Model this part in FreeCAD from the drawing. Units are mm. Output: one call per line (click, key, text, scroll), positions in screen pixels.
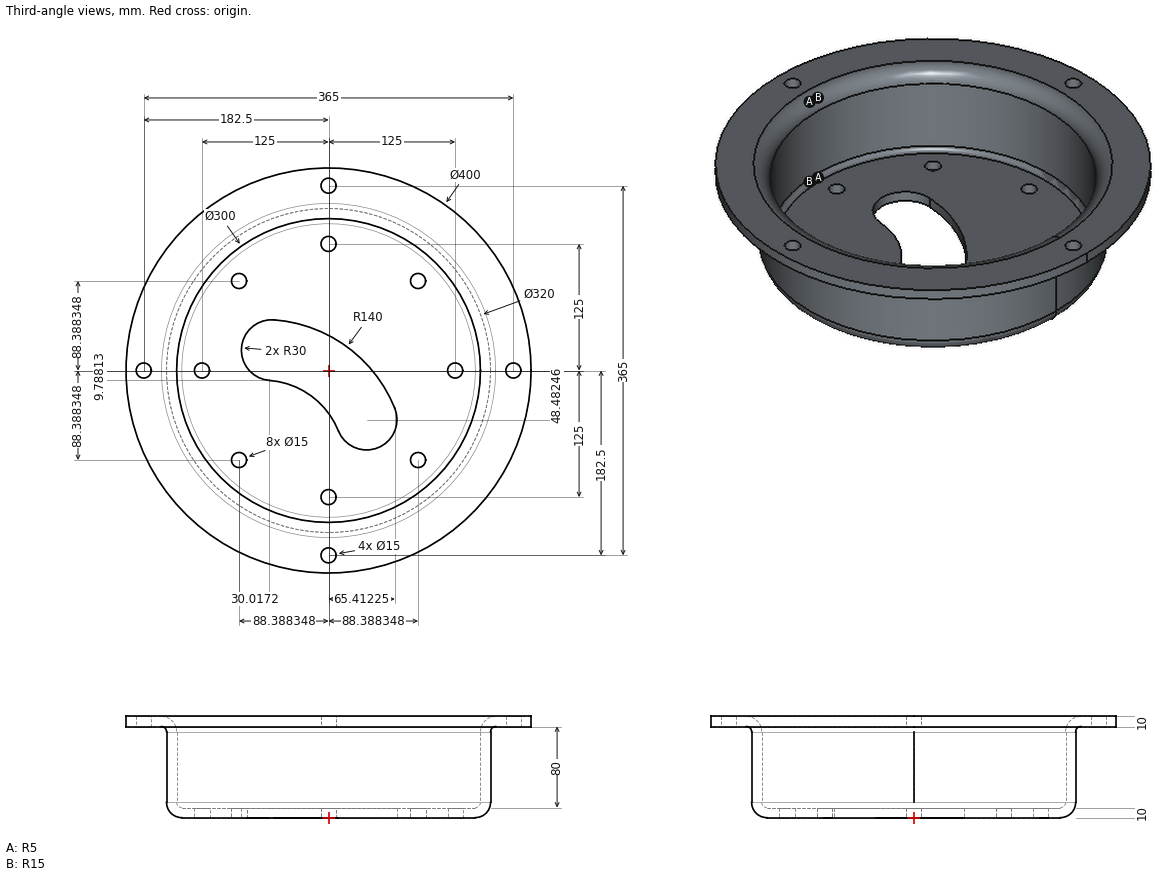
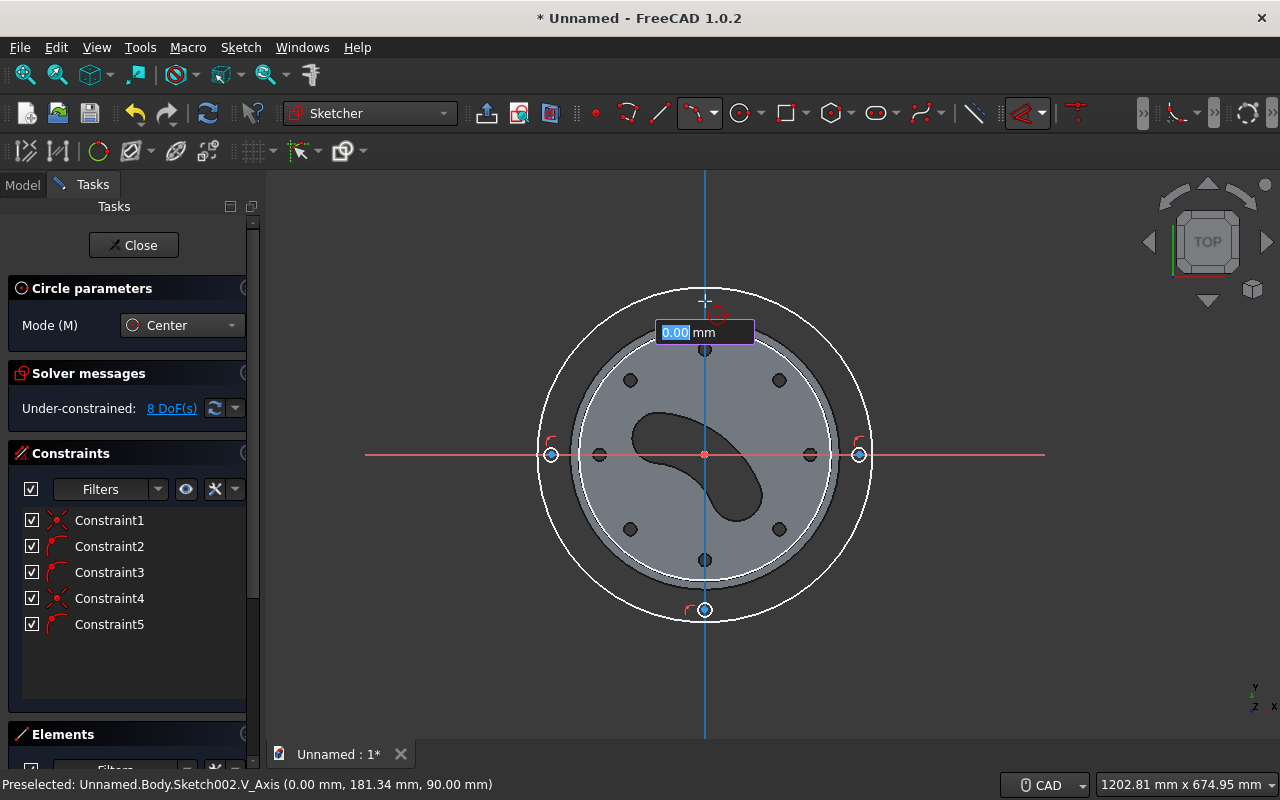
scroll(711, 299, up, 5)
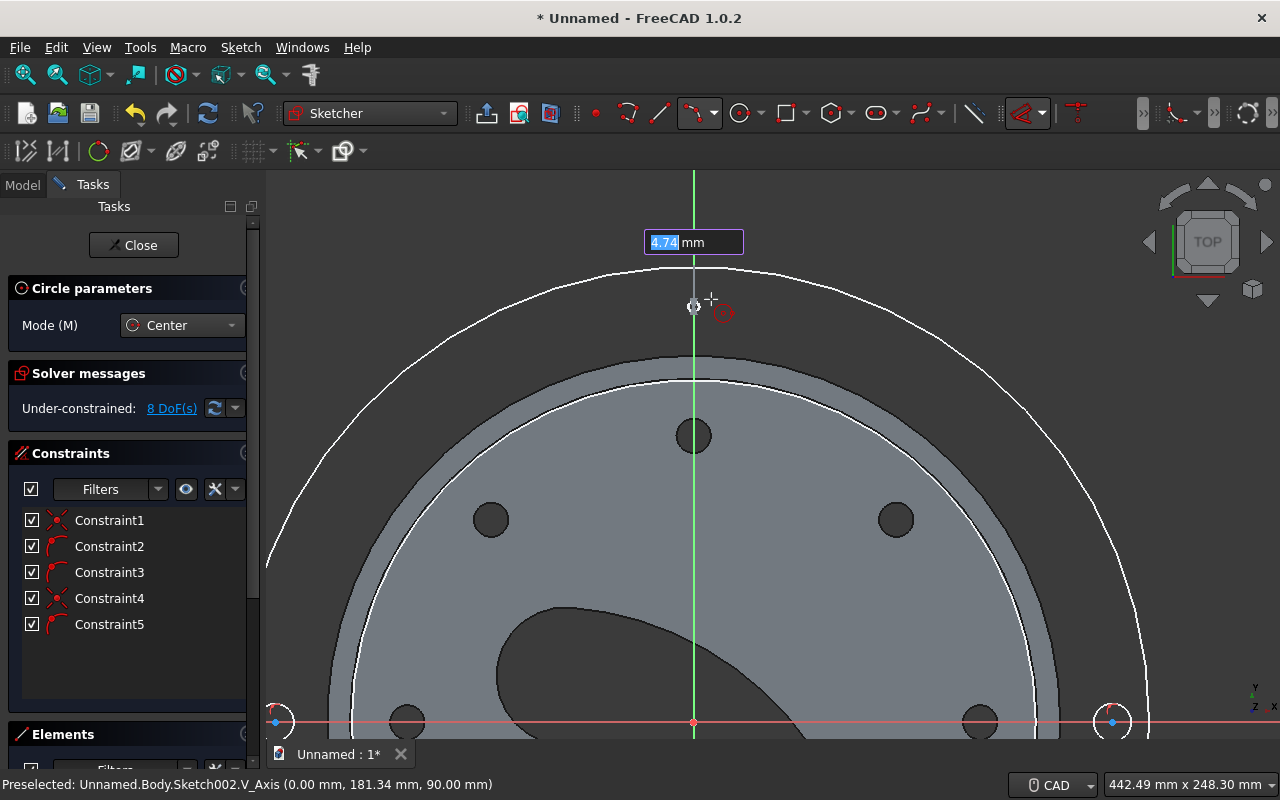
click(710, 298)
key(Escape)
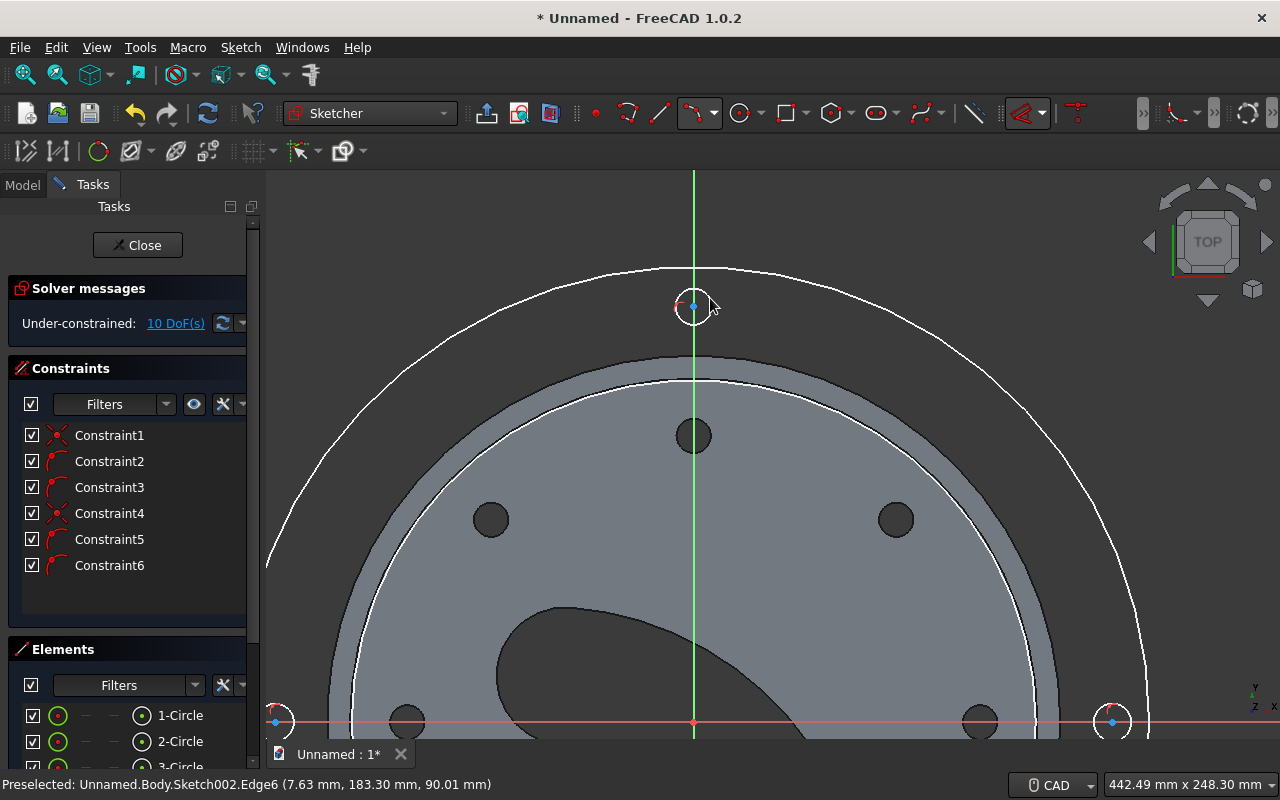
scroll(711, 299, down, 5)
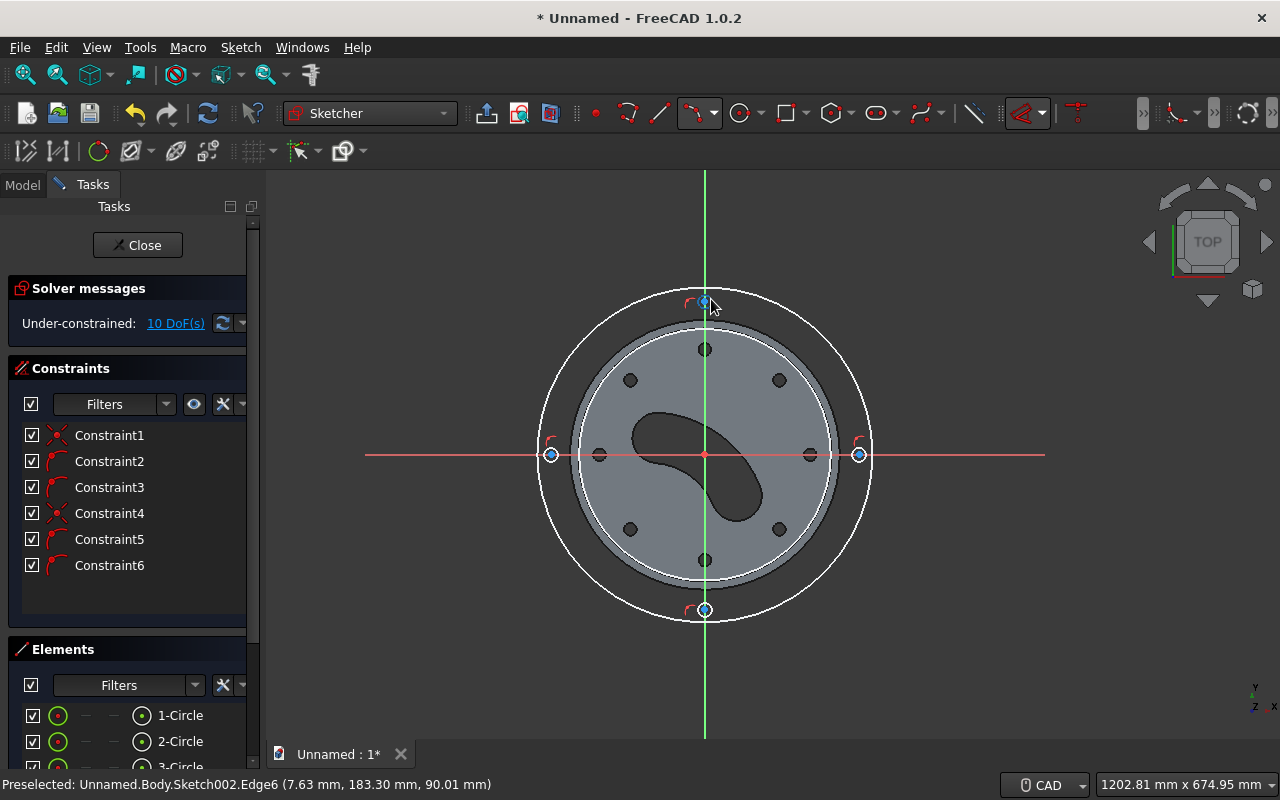
scroll(710, 605, up, 6)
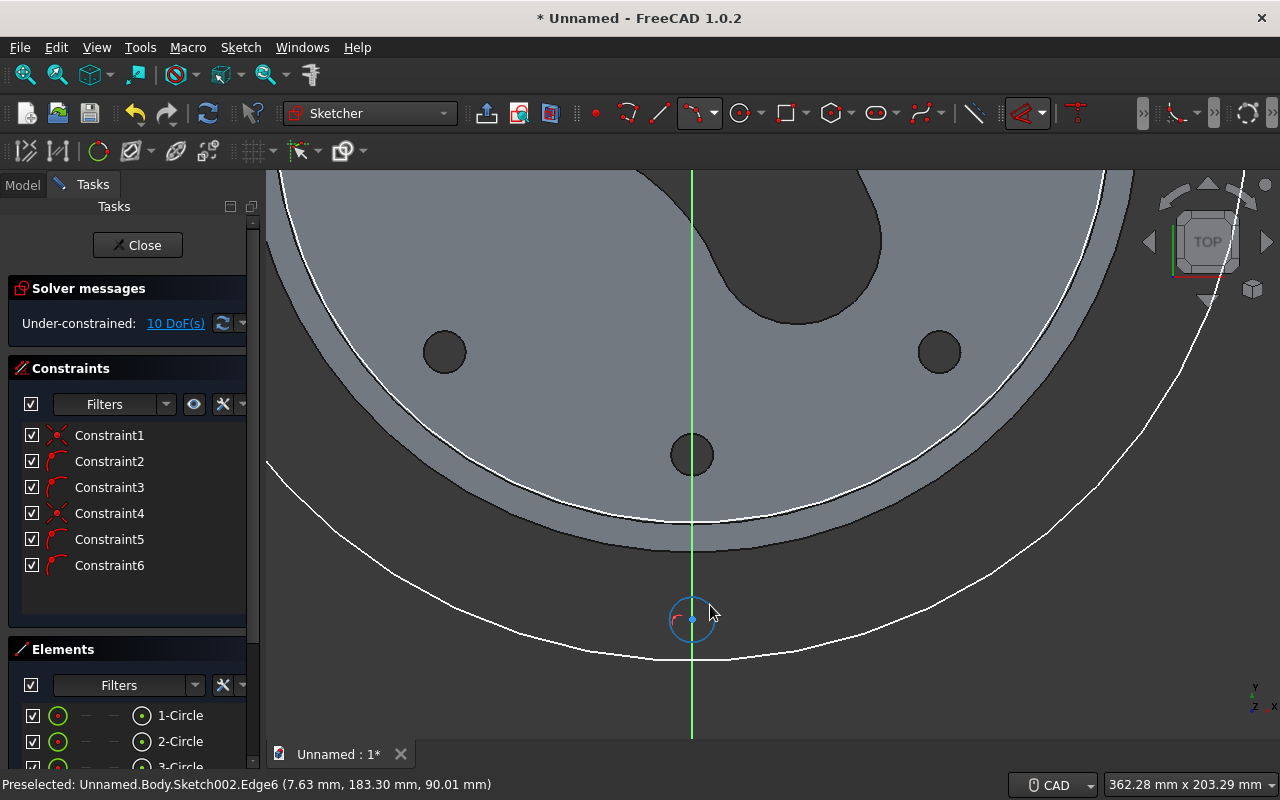
click(708, 604)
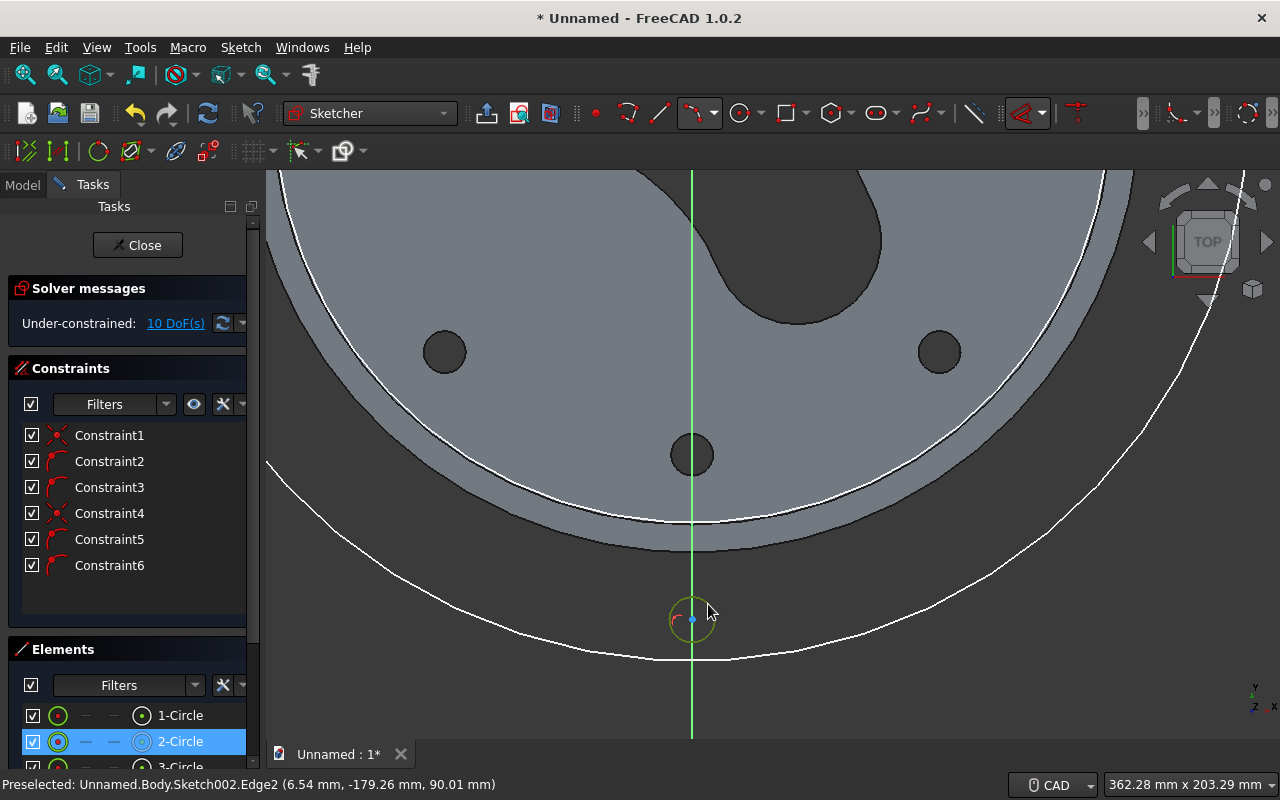
scroll(710, 605, down, 6)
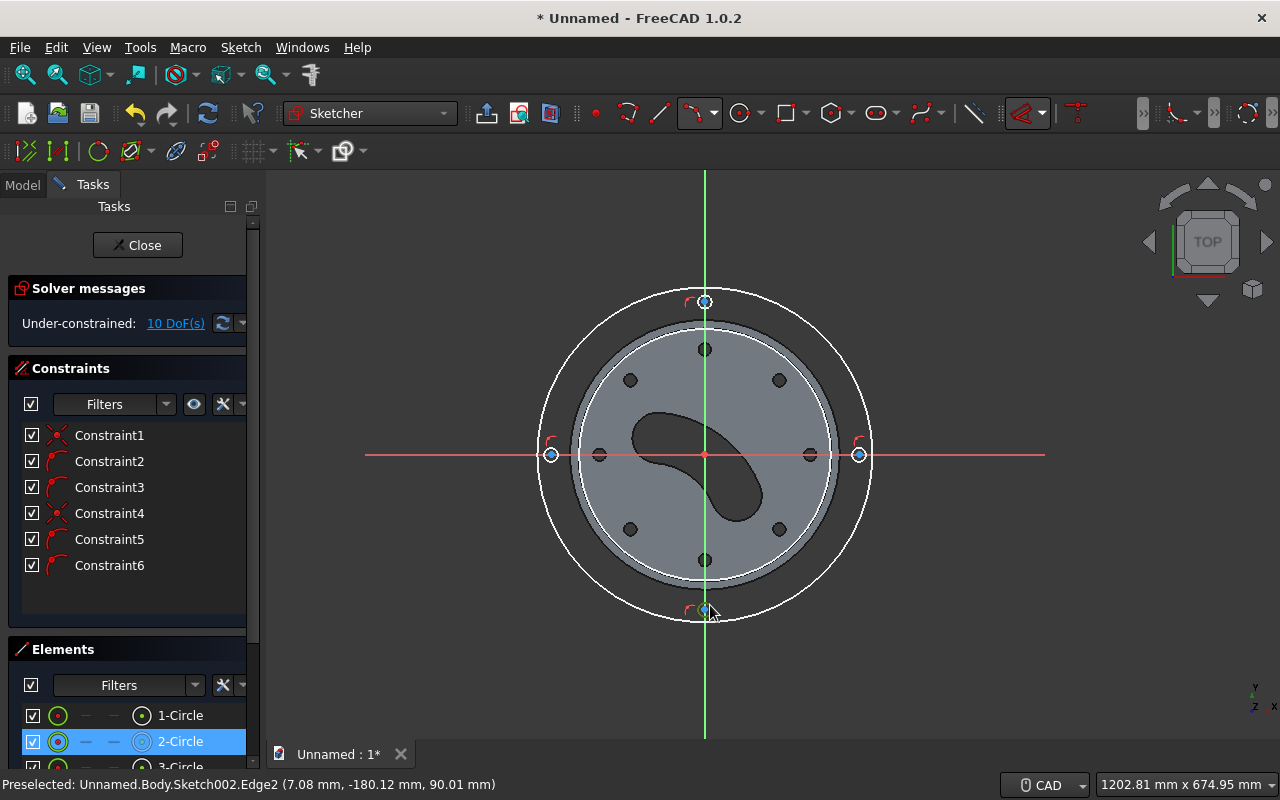
scroll(556, 450, up, 6)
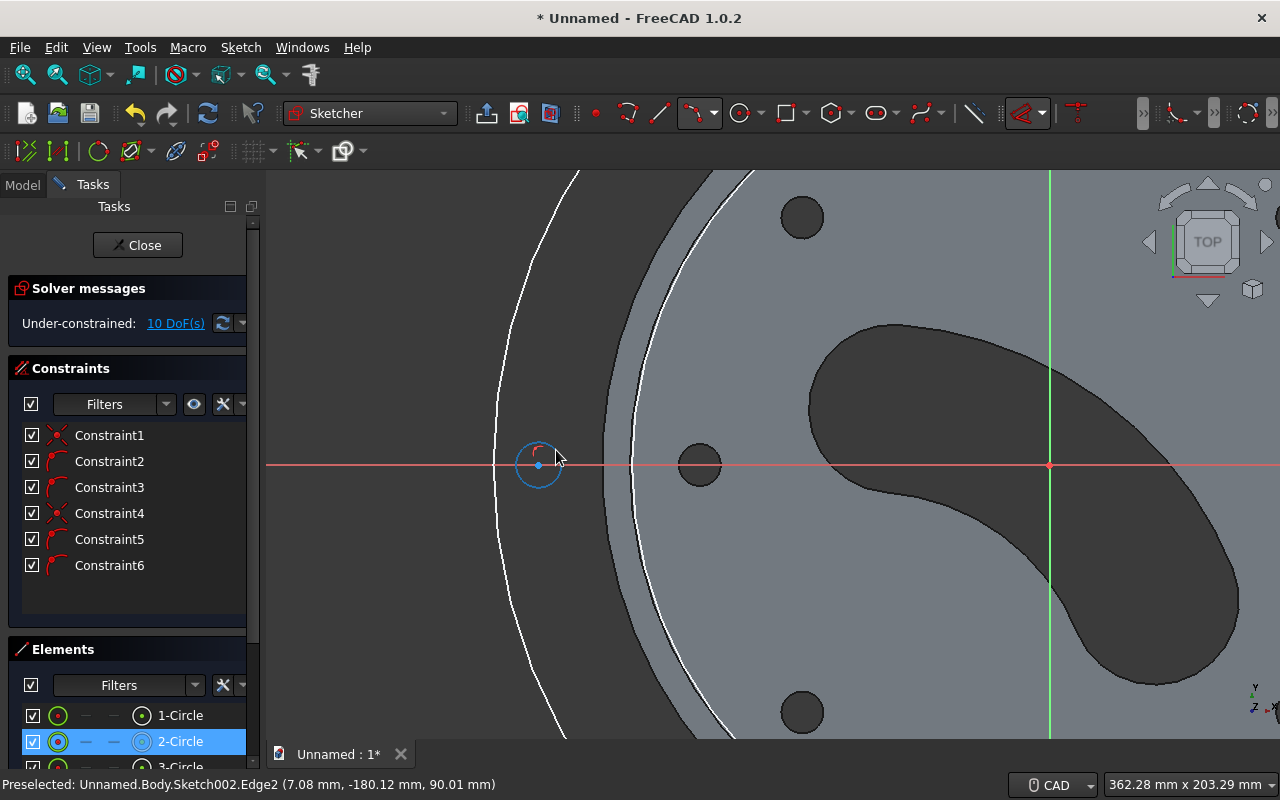
click(555, 449)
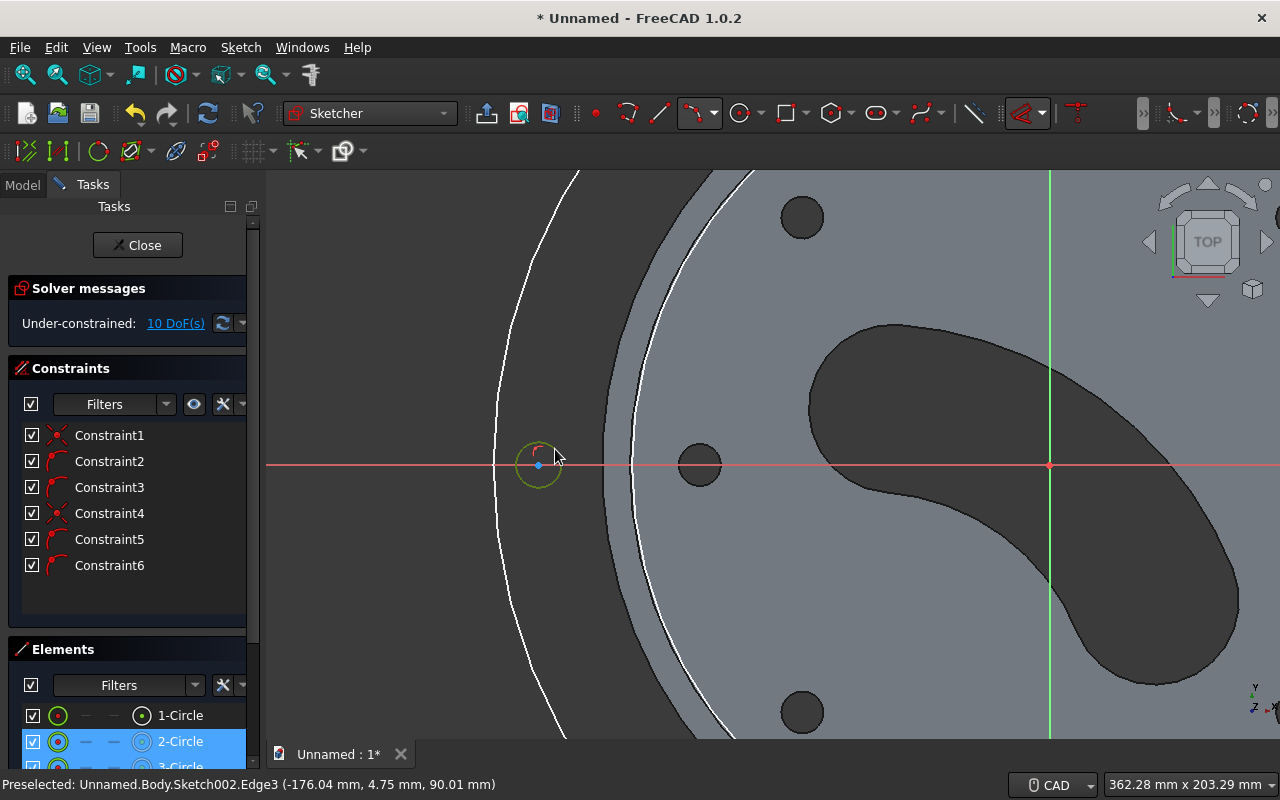
scroll(556, 450, down, 6)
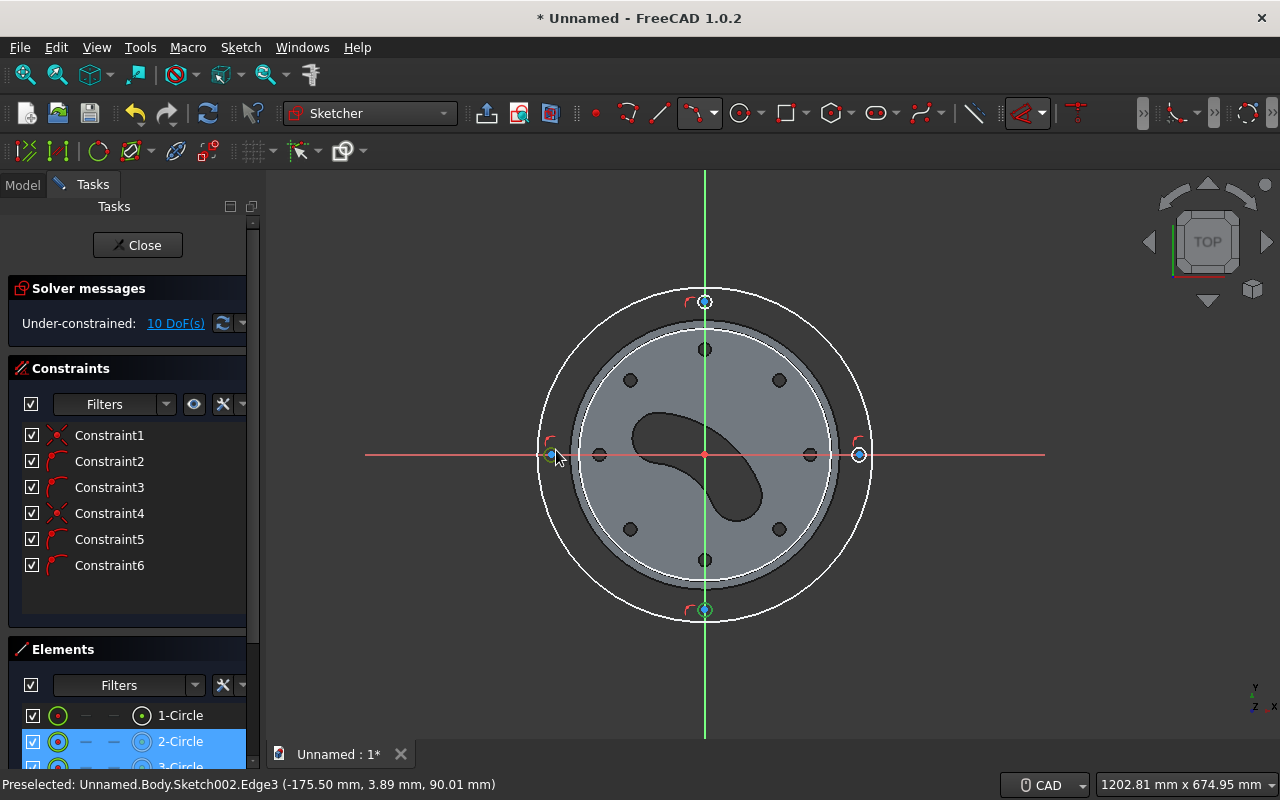
scroll(864, 450, up, 6)